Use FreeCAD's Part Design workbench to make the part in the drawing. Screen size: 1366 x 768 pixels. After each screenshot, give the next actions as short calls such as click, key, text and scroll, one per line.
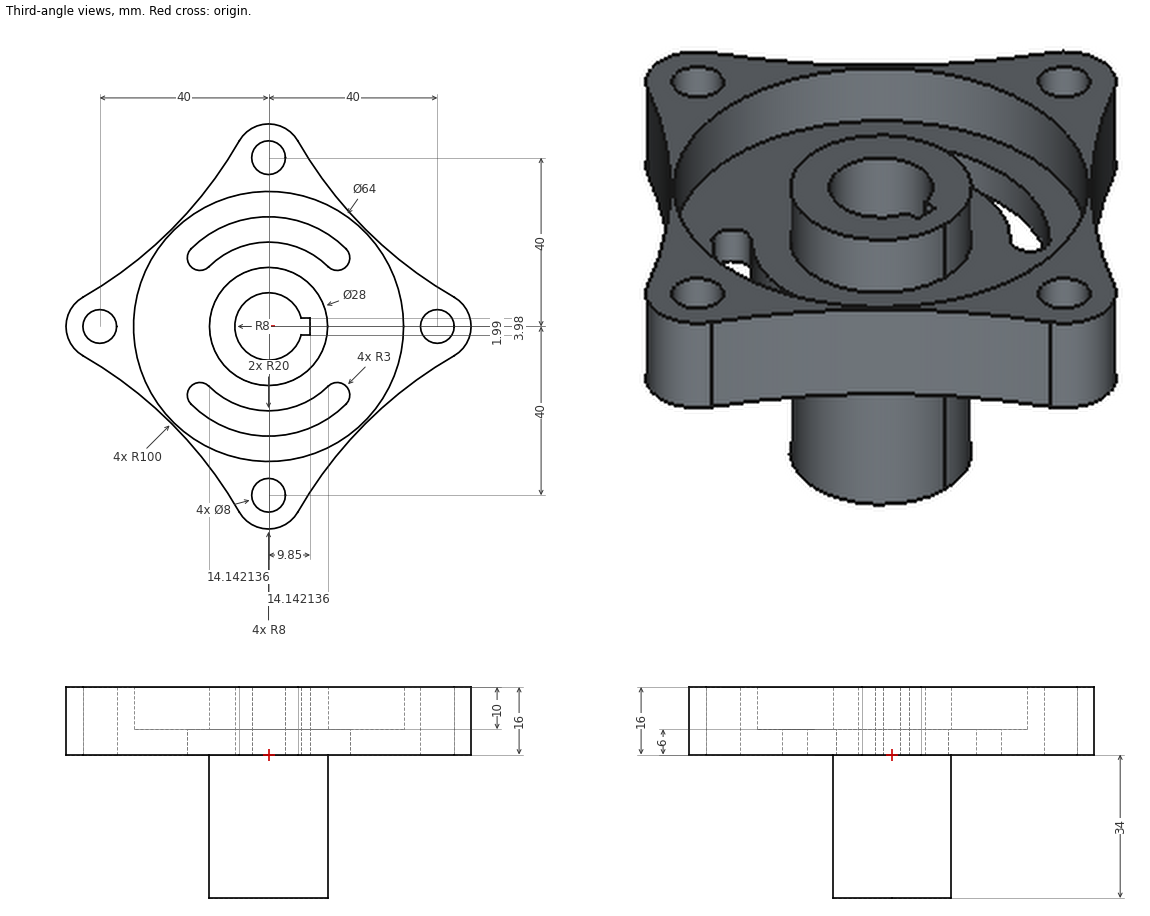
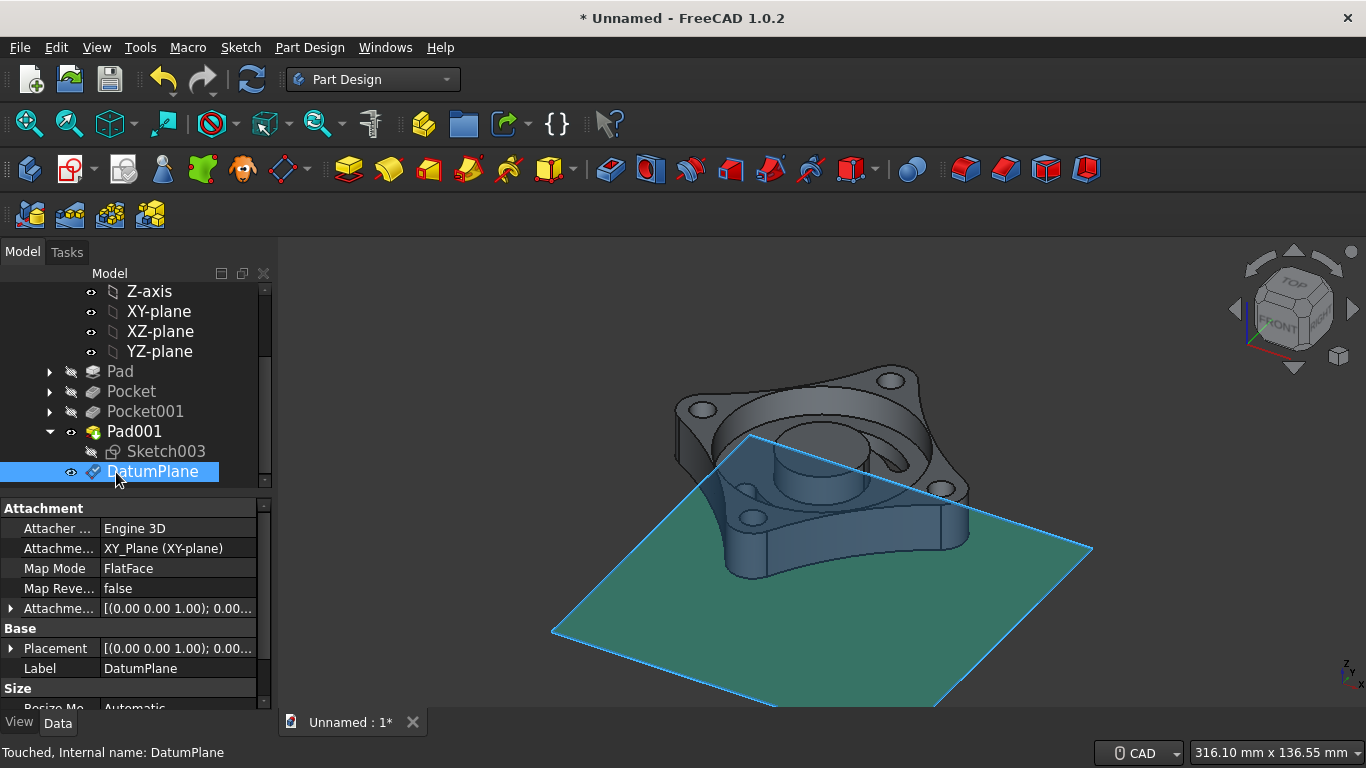
click(70, 170)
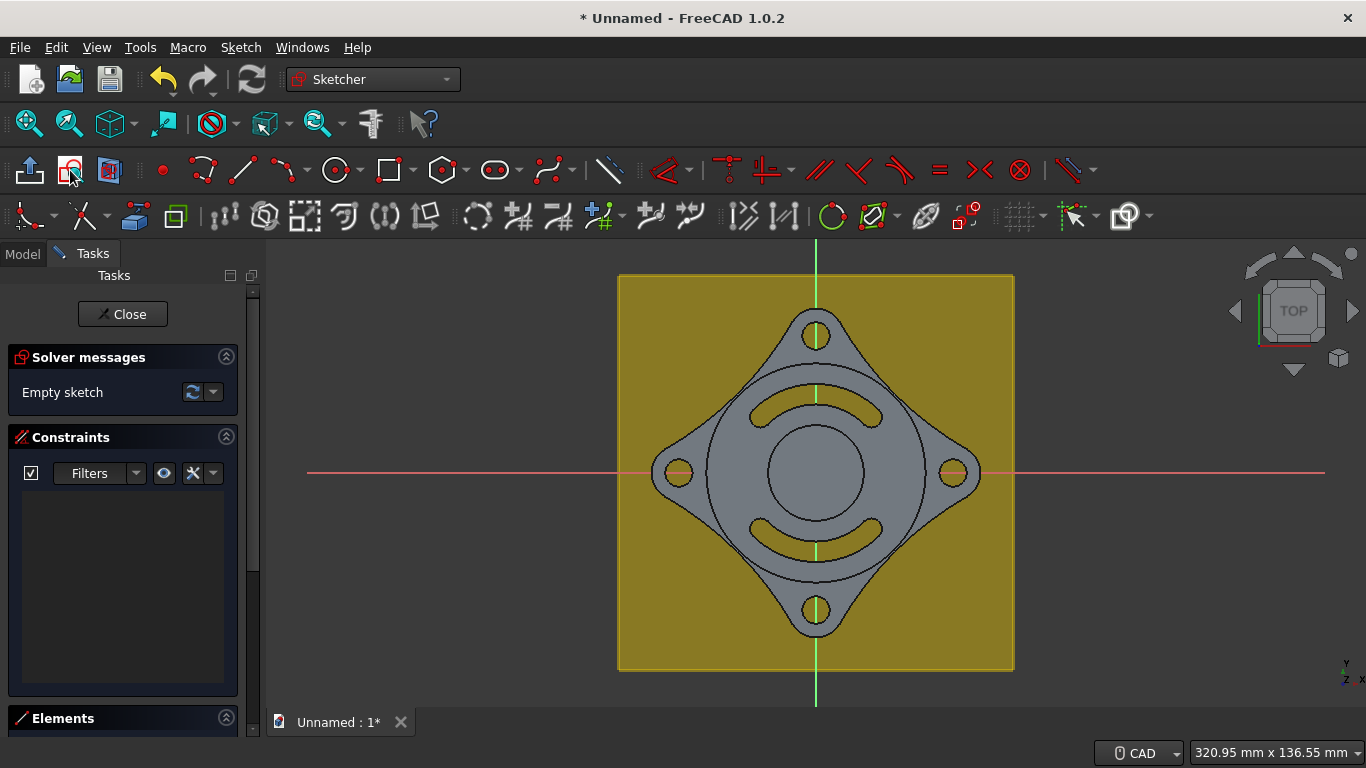
click(110, 170)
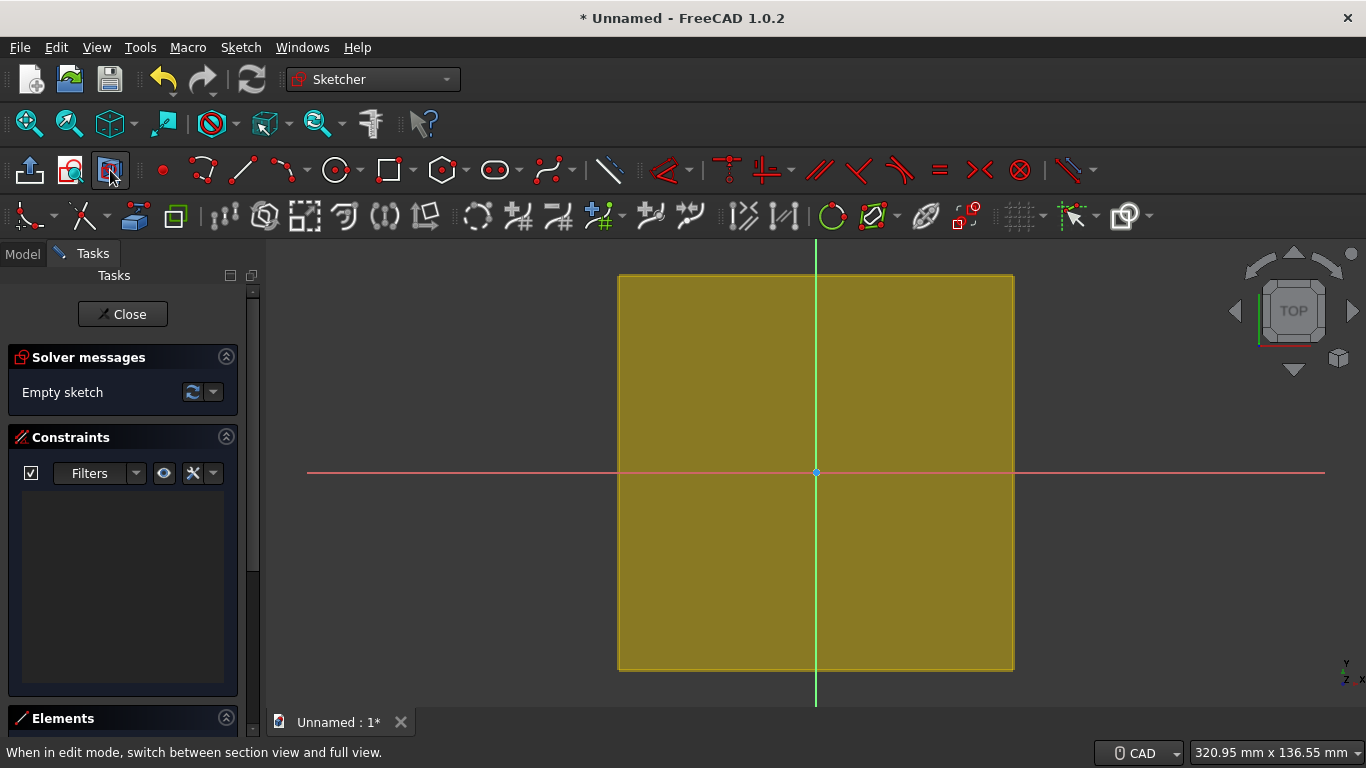
scroll(846, 473, up, 6)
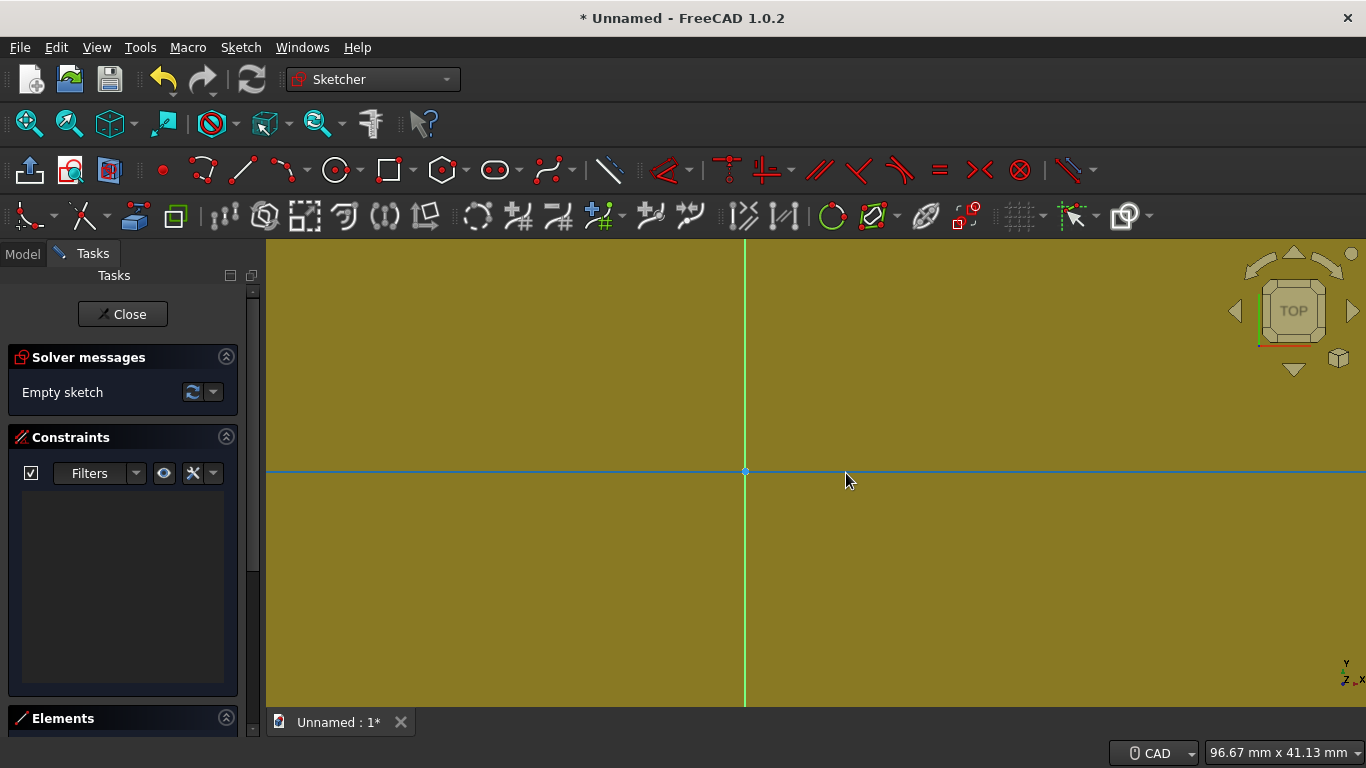
click(336, 170)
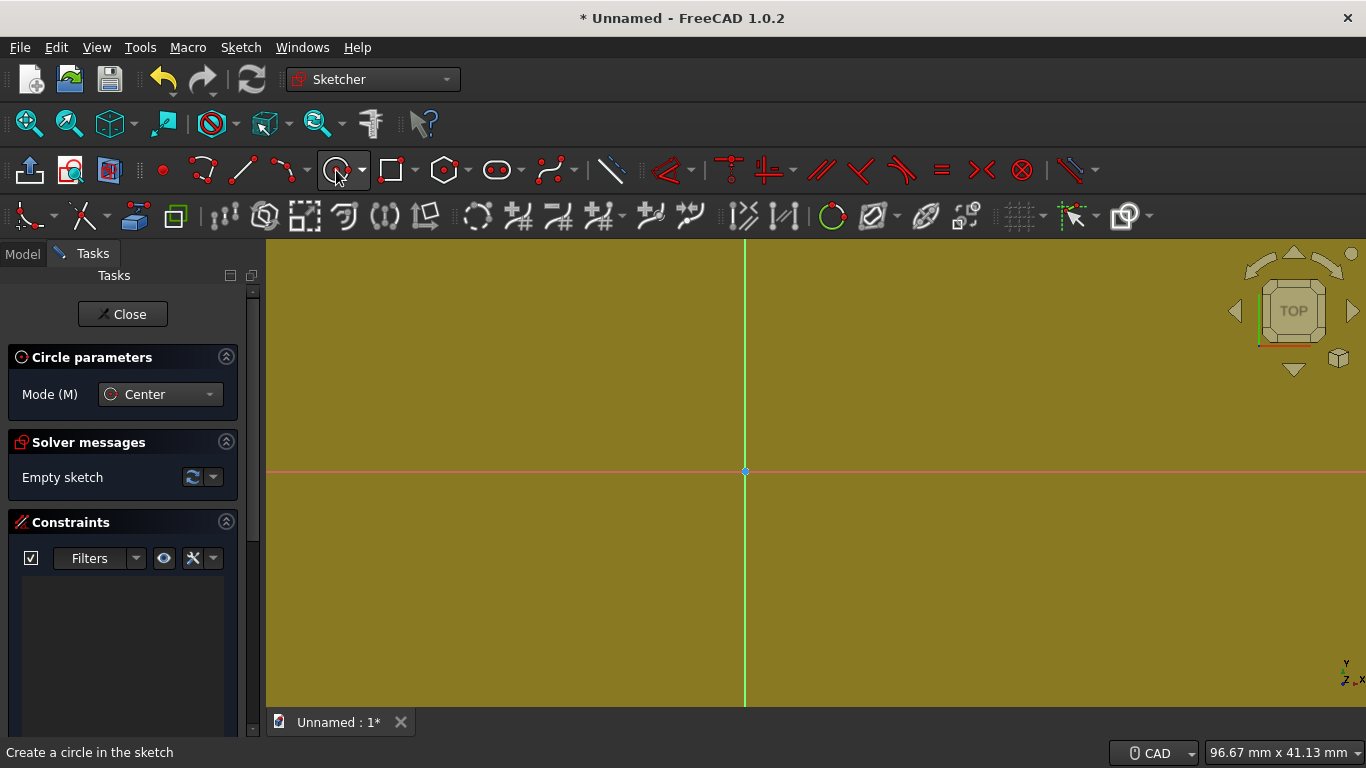
click(745, 472)
move(858, 359)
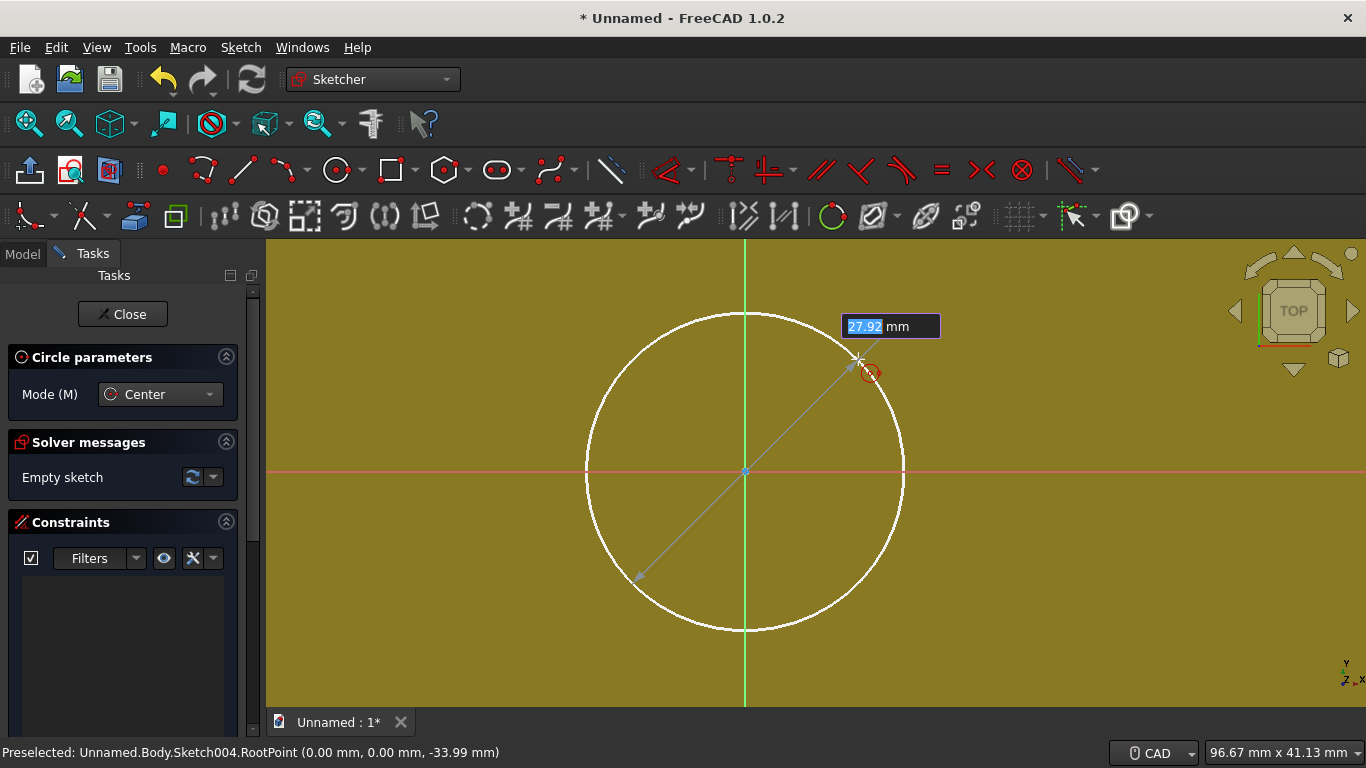
text(28)
key(Return)
key(Escape)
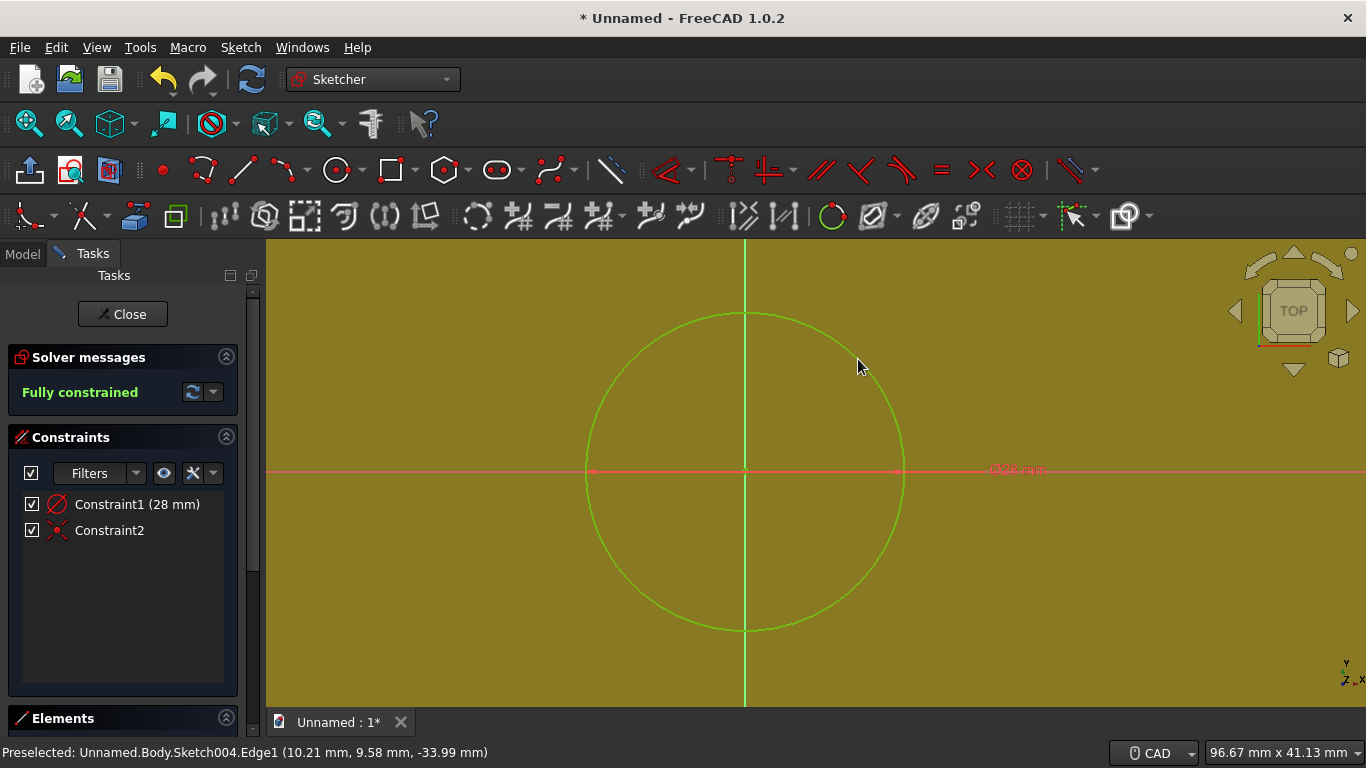
click(123, 314)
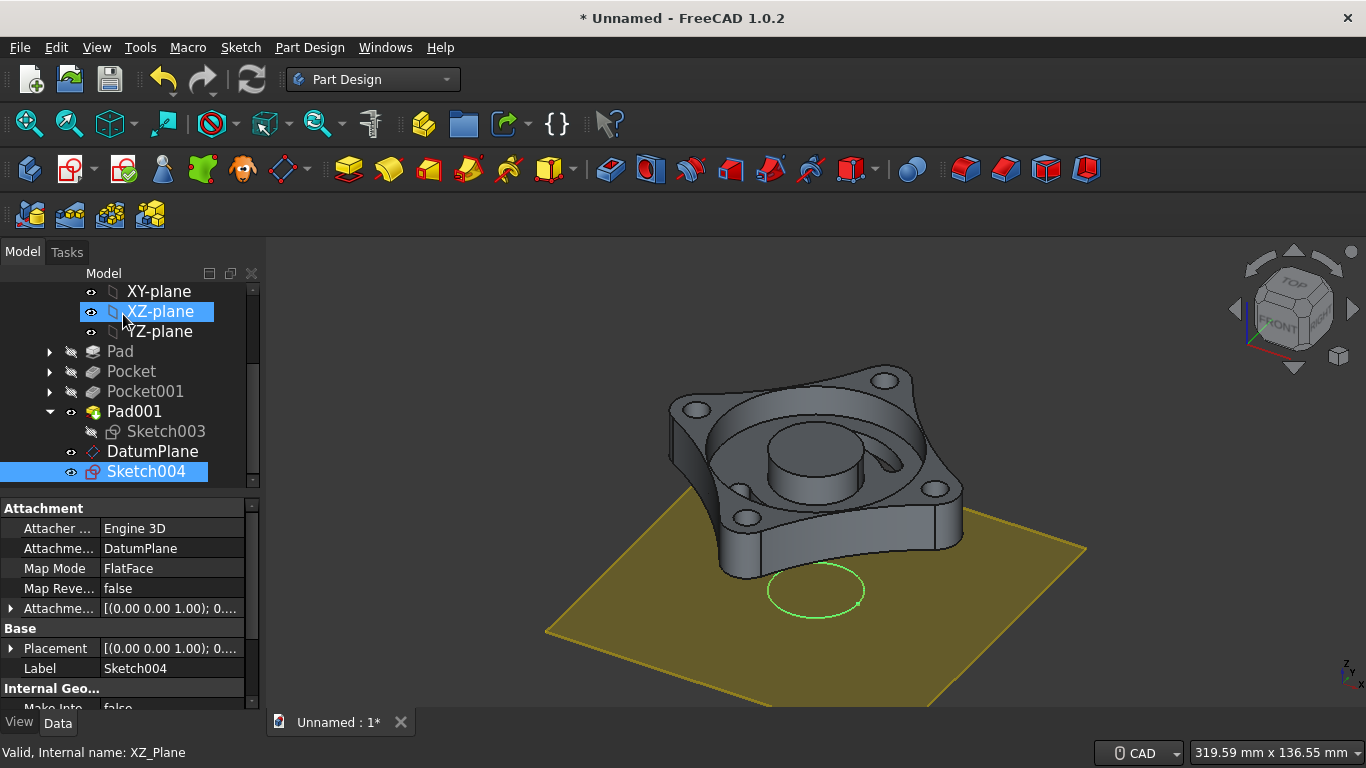
click(350, 170)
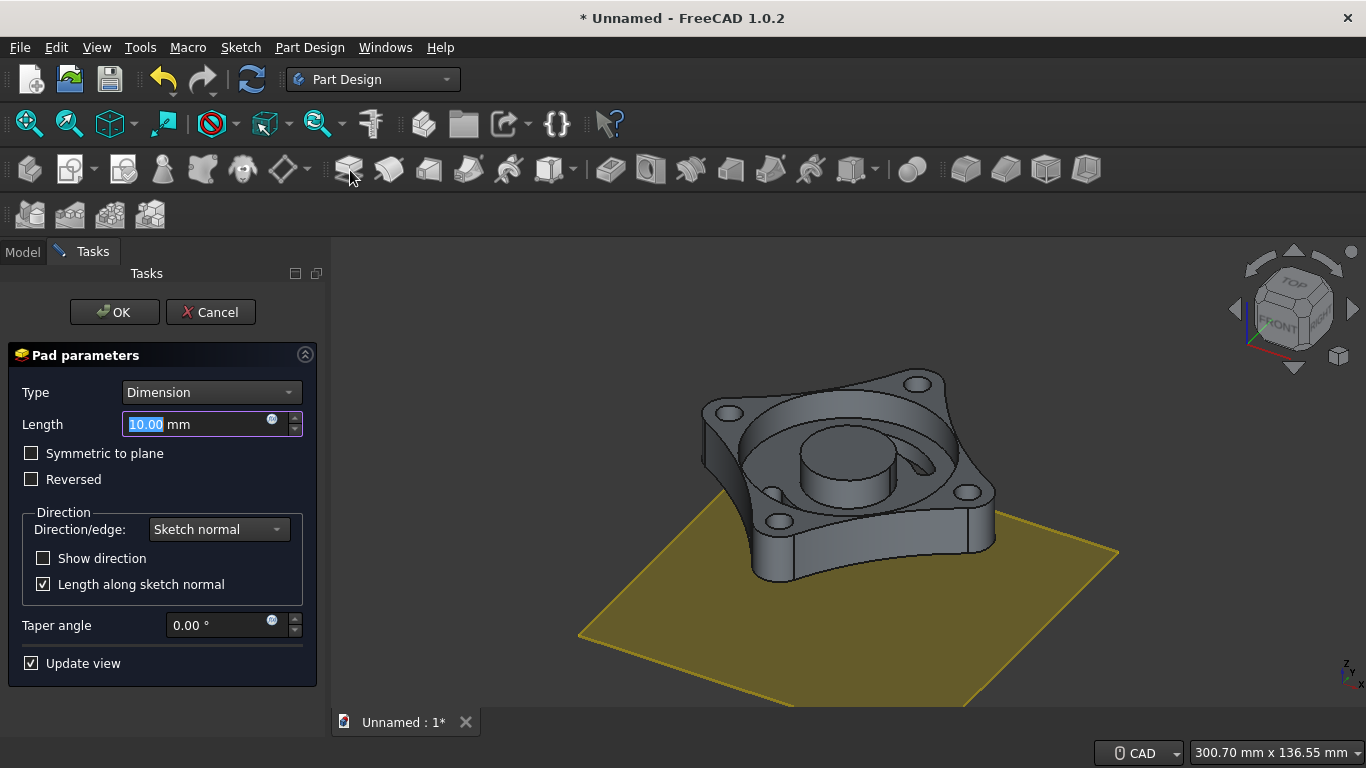
text(34)
key(Tab)